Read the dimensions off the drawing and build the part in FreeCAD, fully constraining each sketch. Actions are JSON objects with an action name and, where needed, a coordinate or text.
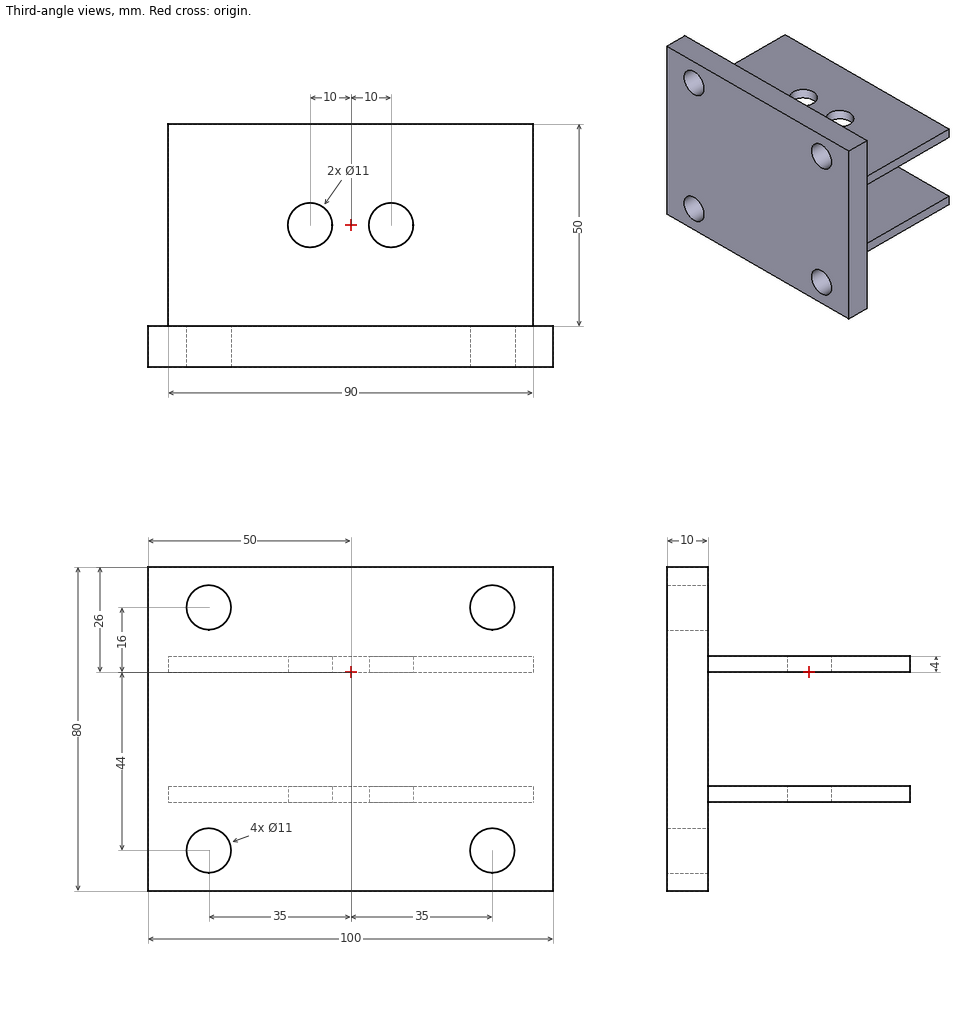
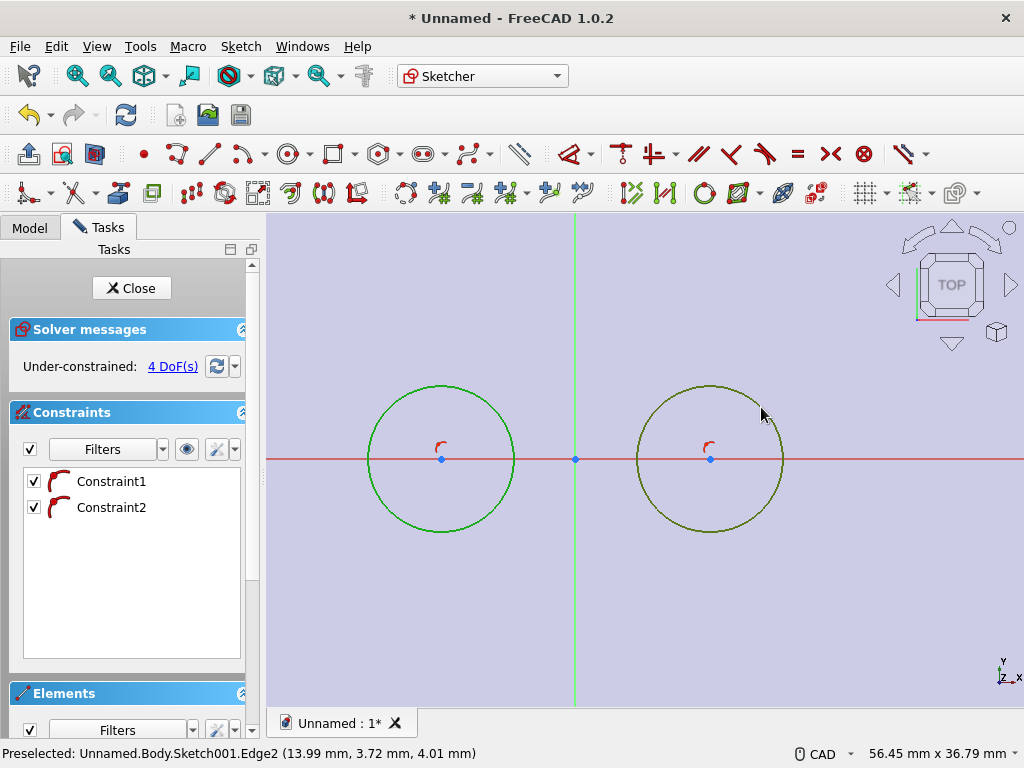
{"action": "key", "text": "e"}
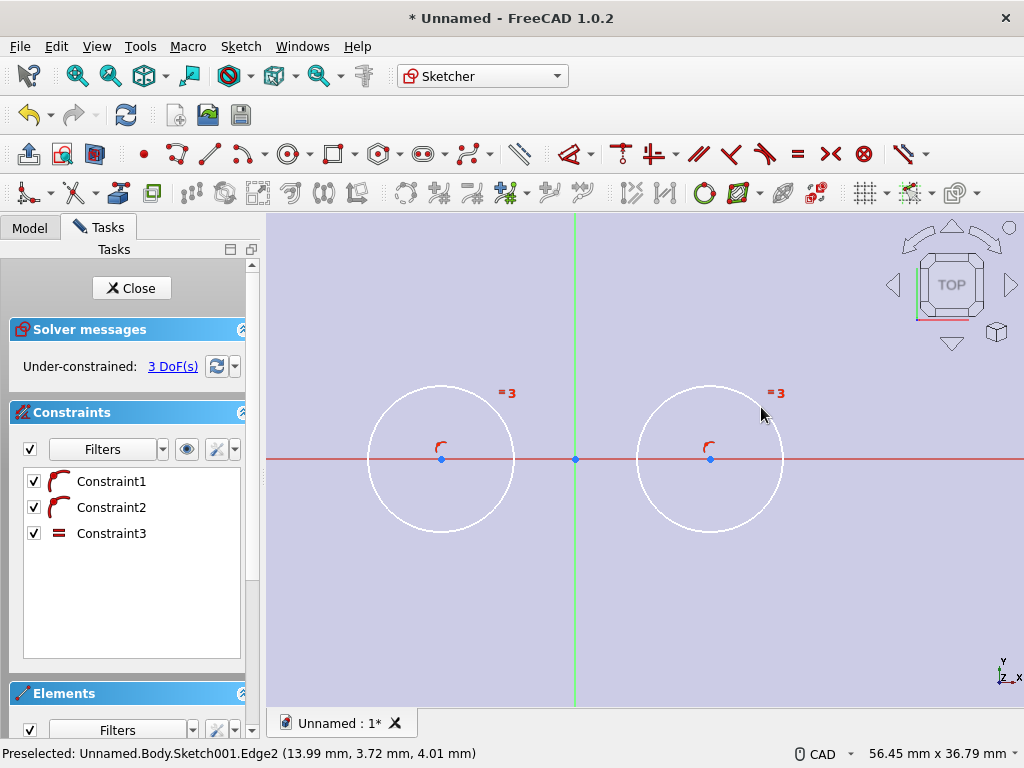
{"action": "left_click", "coordinate": [568, 154]}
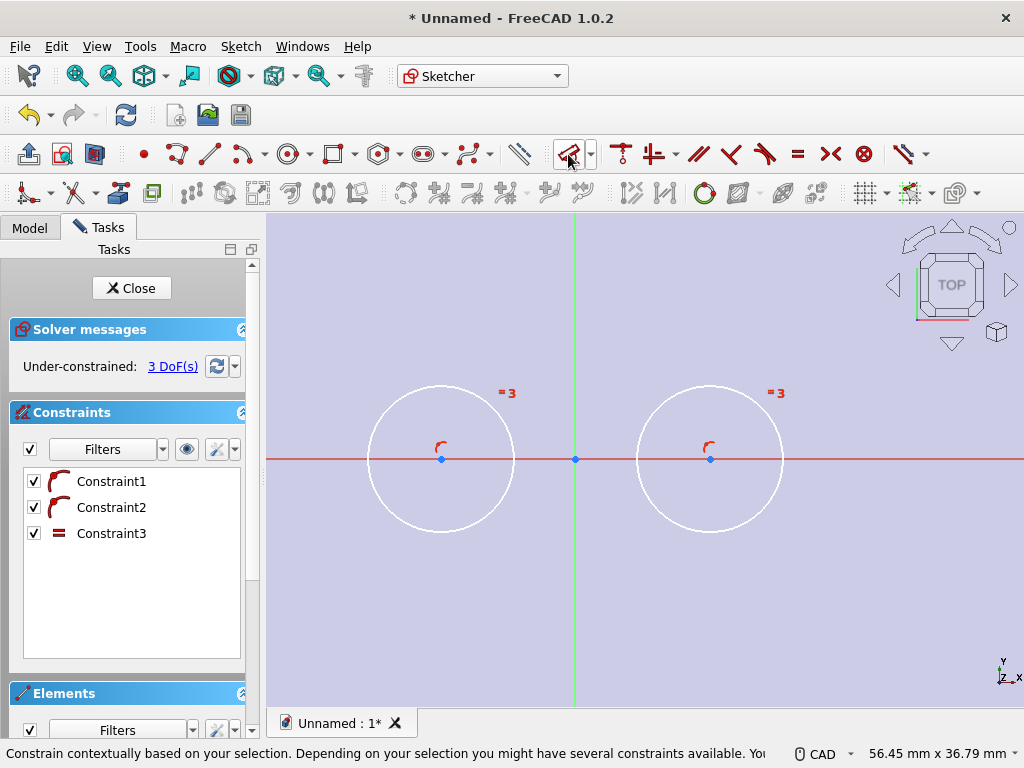
{"action": "left_click", "coordinate": [492, 407]}
{"action": "left_click", "coordinate": [514, 384]}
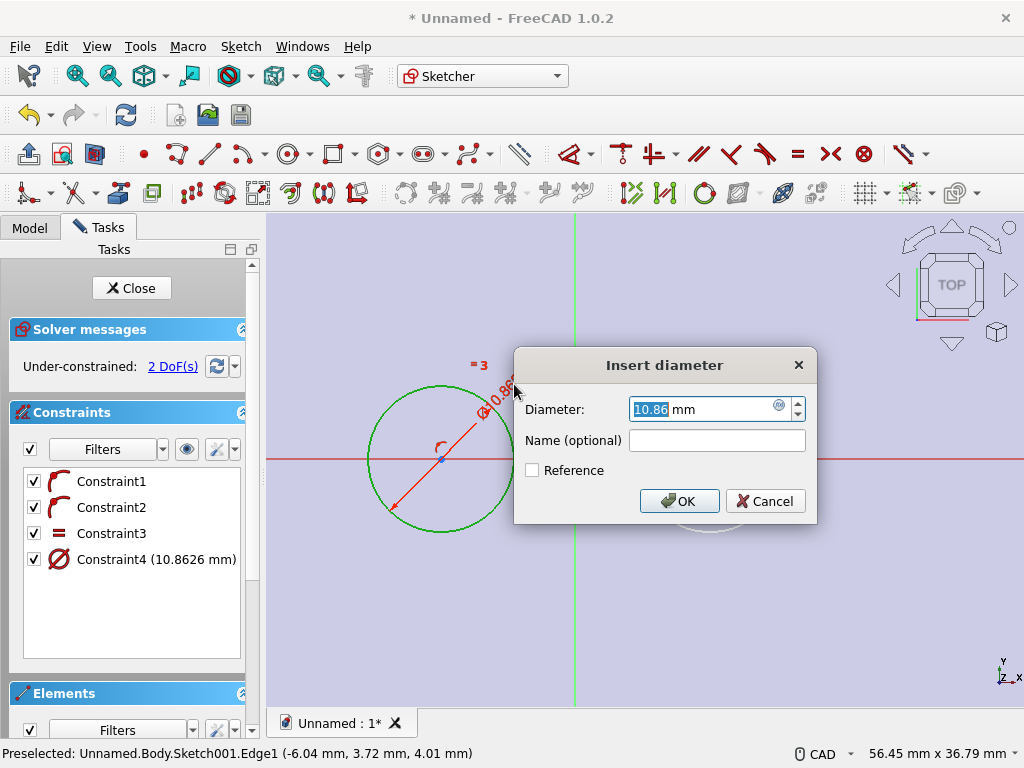
{"action": "type", "text": "11"}
{"action": "key", "text": "Return"}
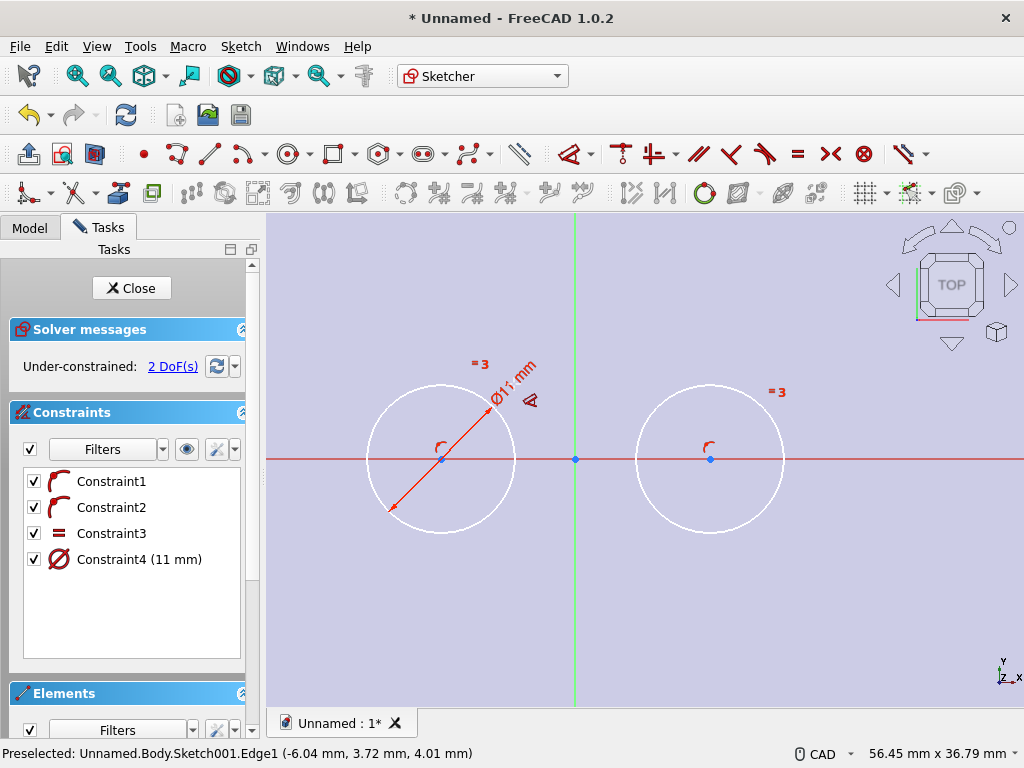
{"action": "left_click", "coordinate": [441, 459]}
{"action": "left_click", "coordinate": [477, 493]}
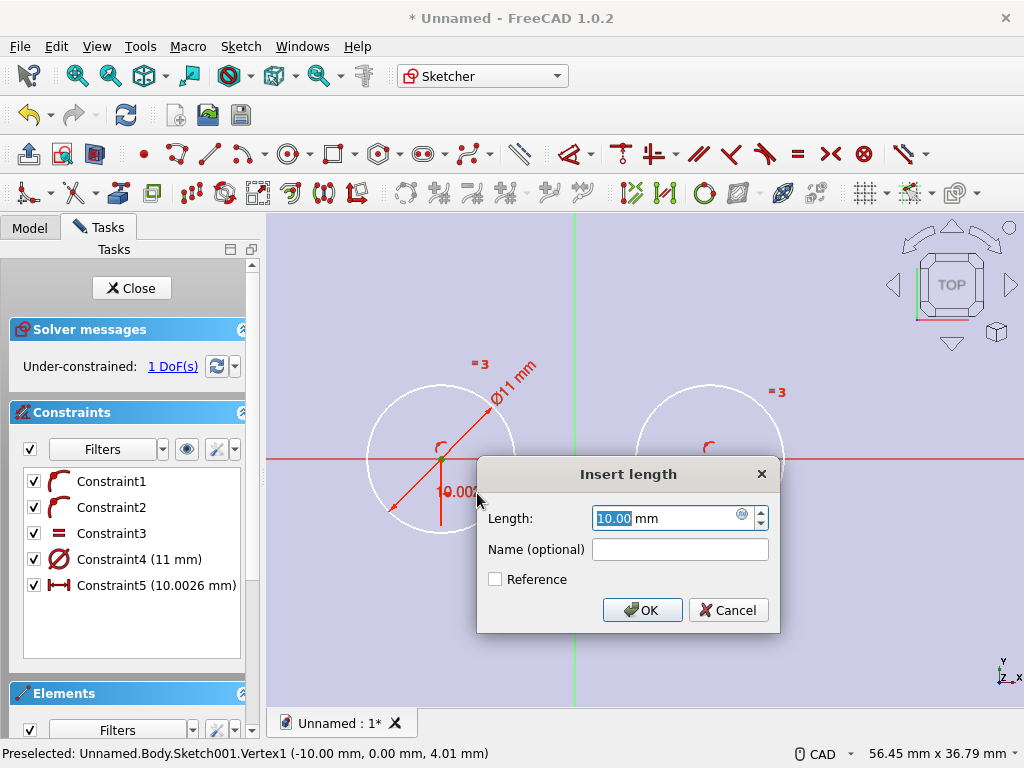
{"action": "type", "text": "10"}
{"action": "key", "text": "Return"}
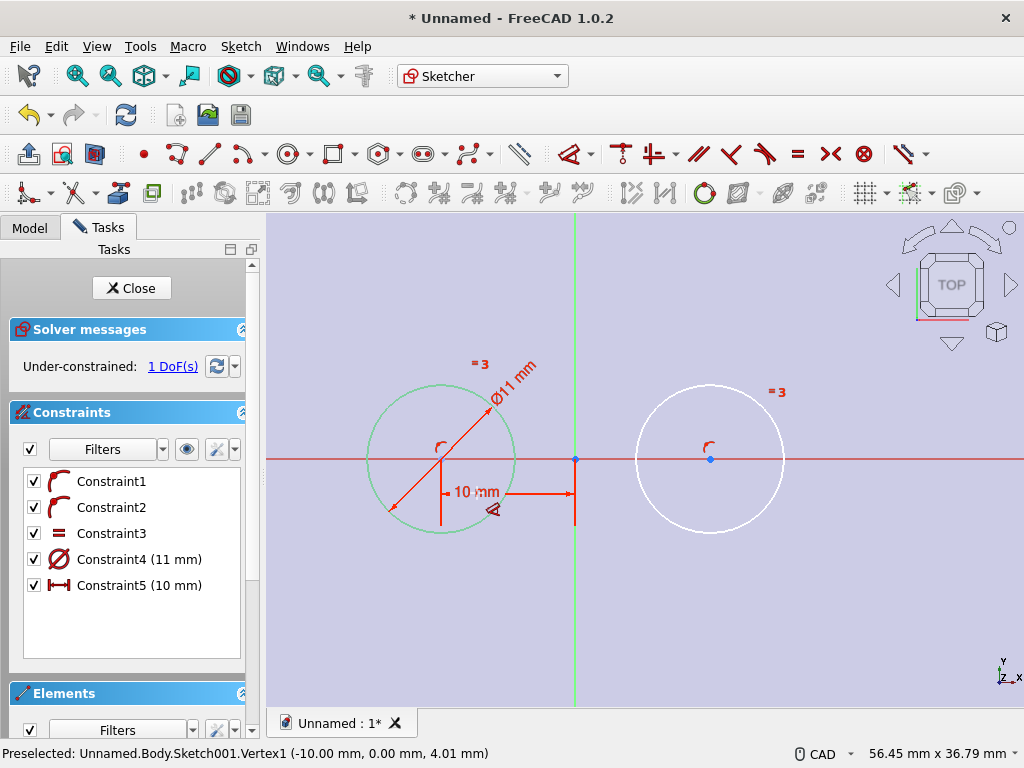
{"action": "left_click", "coordinate": [710, 459]}
{"action": "left_click", "coordinate": [612, 493]}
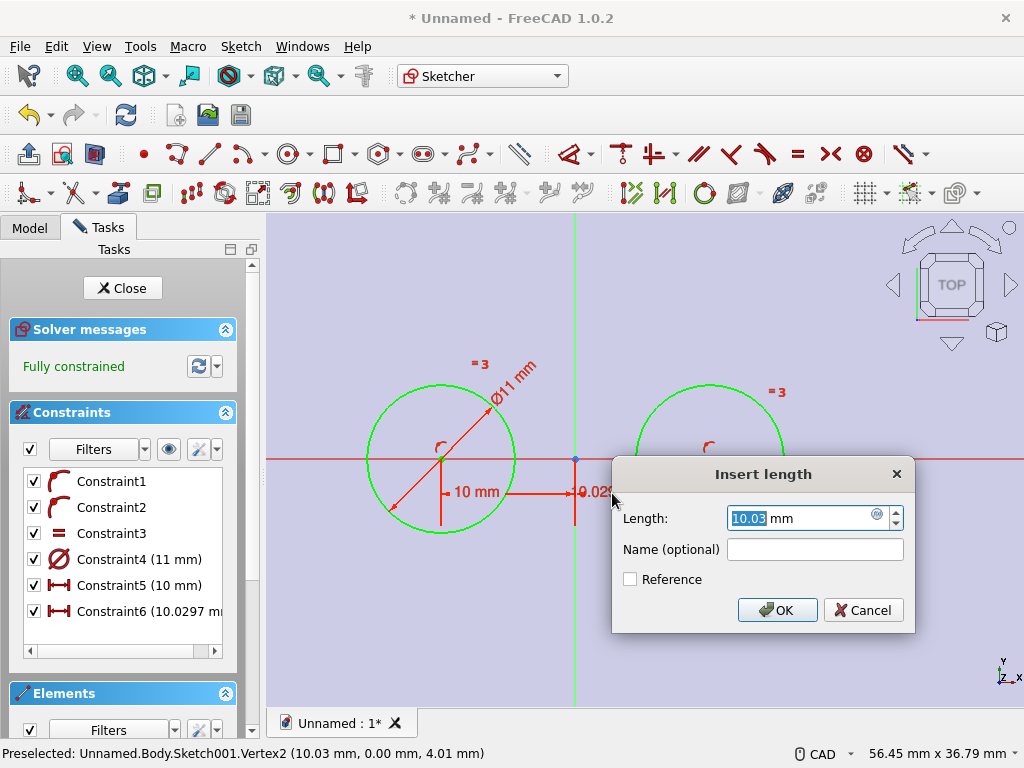
{"action": "type", "text": "10"}
{"action": "key", "text": "Return"}
{"action": "key", "text": "Escape"}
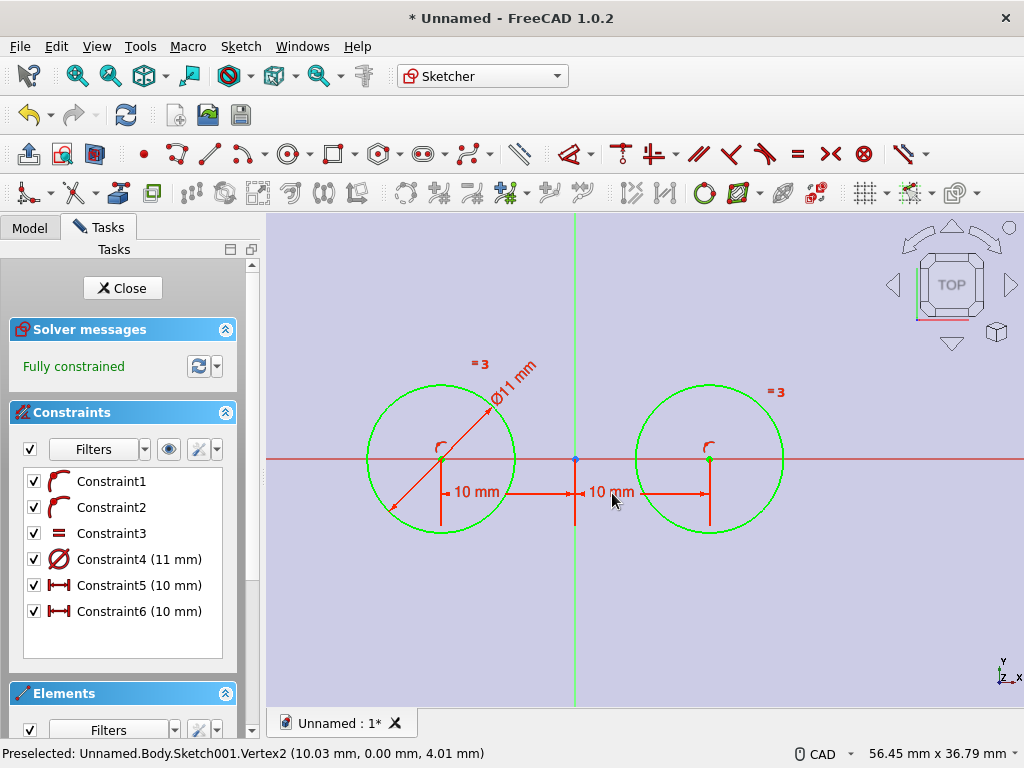
{"action": "left_click", "coordinate": [123, 288]}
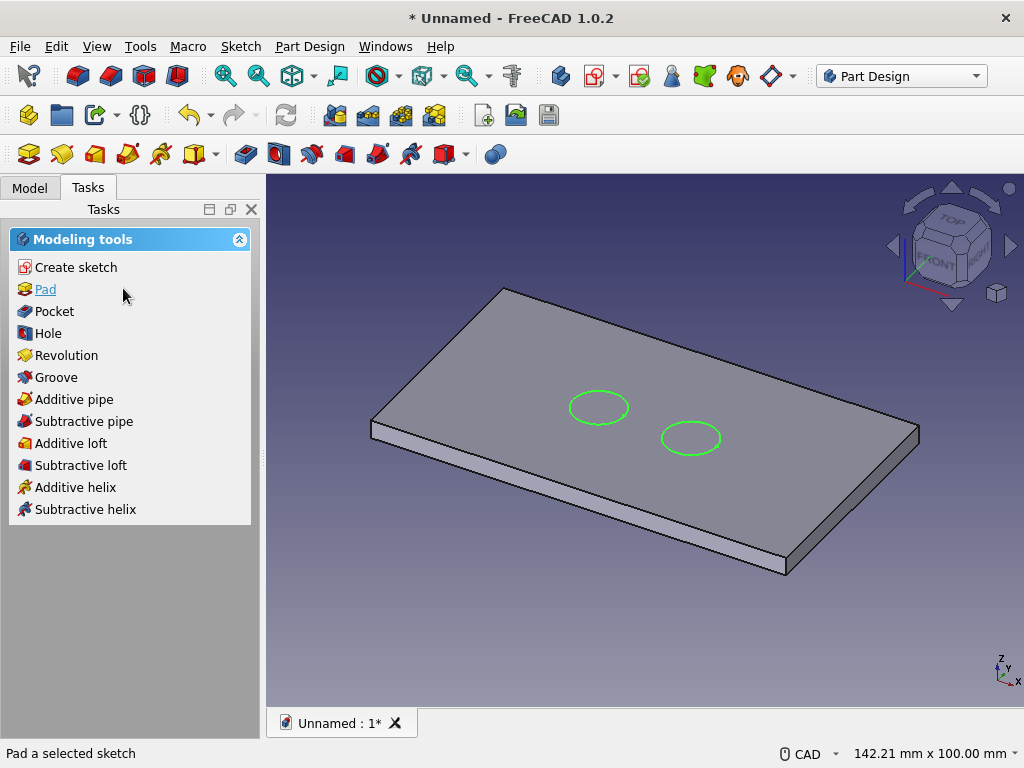
{"action": "left_click", "coordinate": [246, 154]}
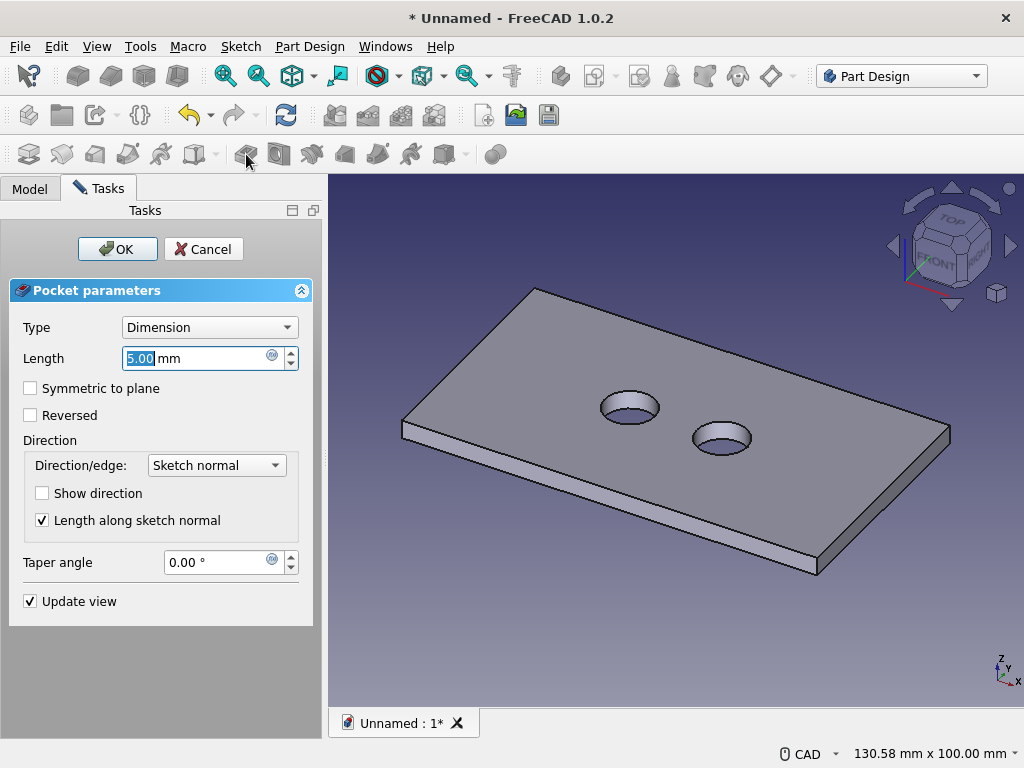
{"action": "left_click", "coordinate": [210, 328]}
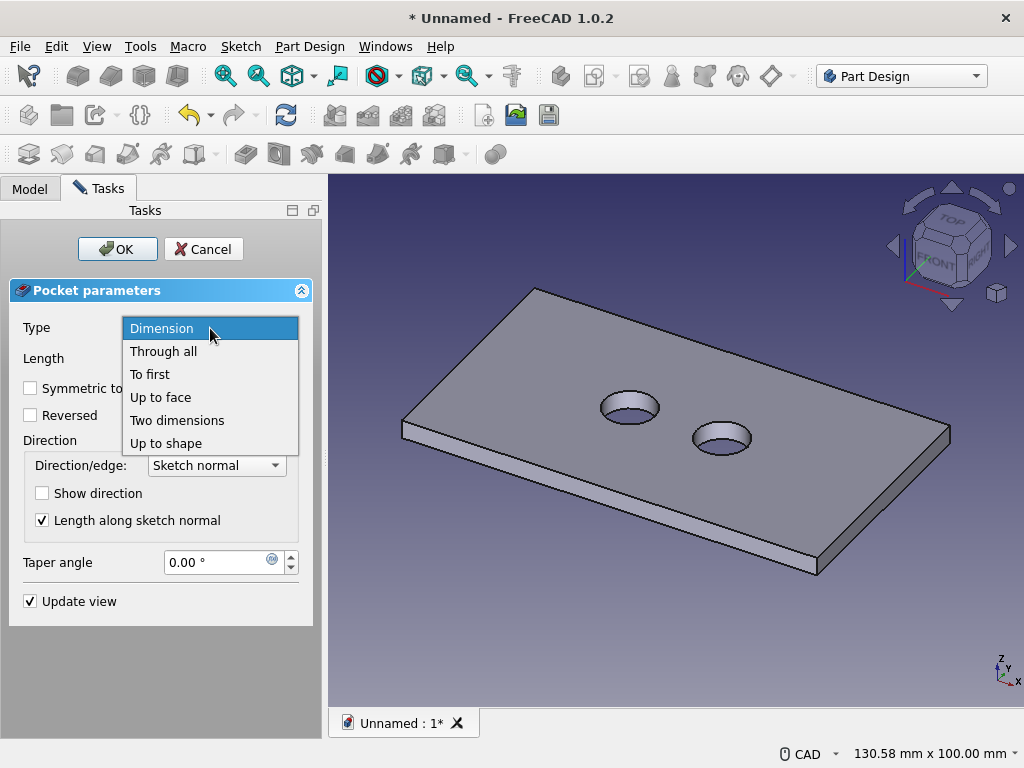
{"action": "left_click", "coordinate": [208, 352]}